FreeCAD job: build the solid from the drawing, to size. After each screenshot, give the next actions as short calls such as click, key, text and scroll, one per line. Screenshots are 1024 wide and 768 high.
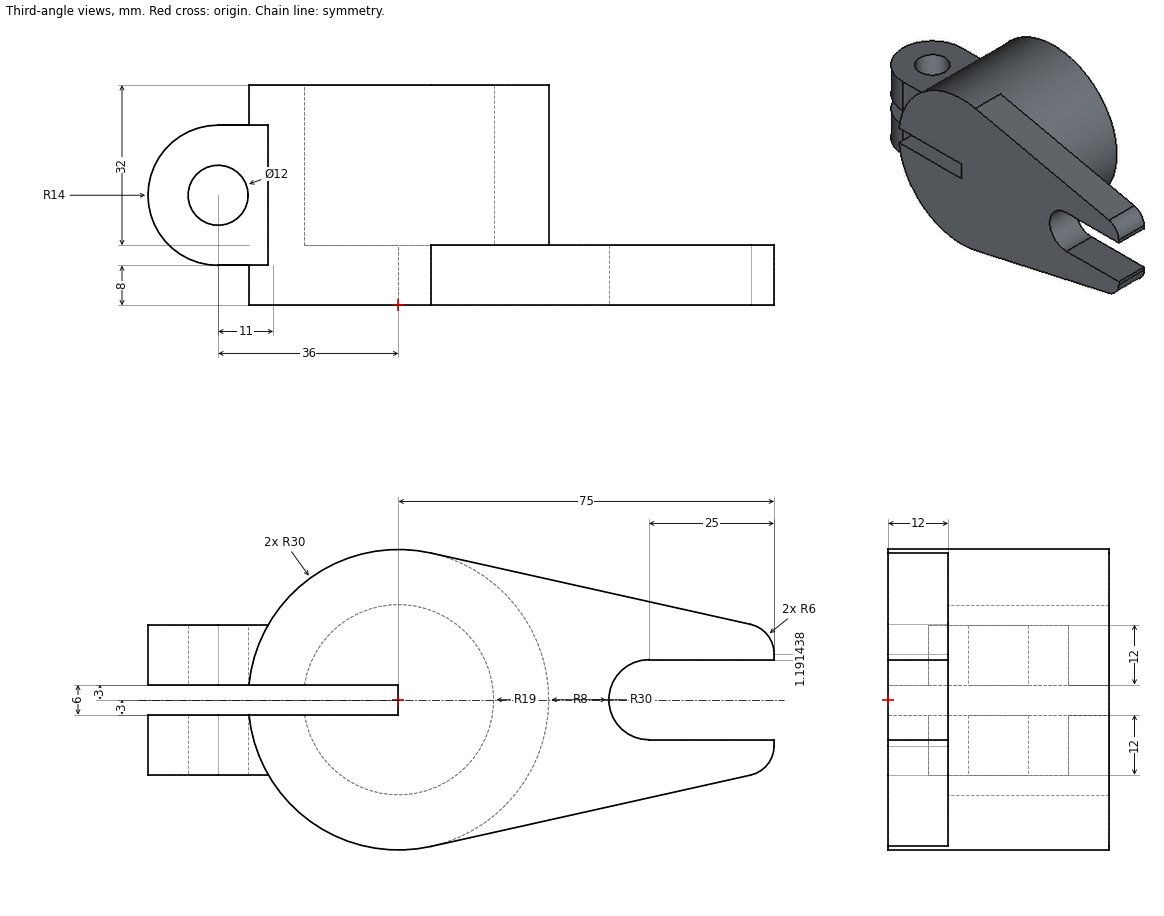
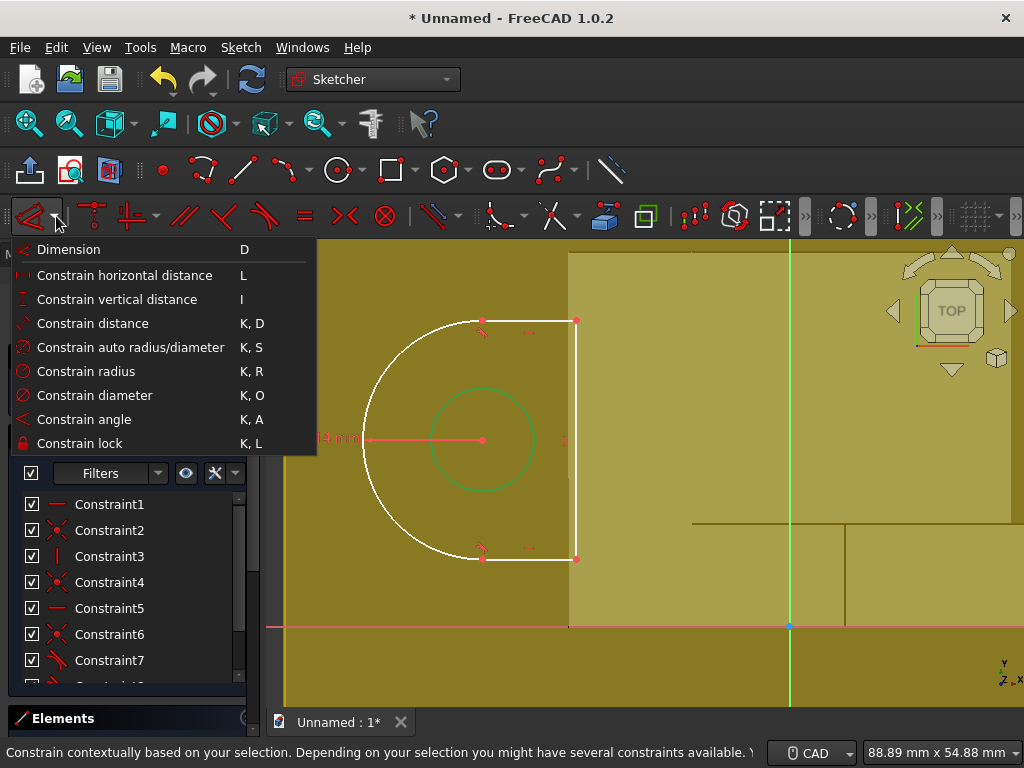
click(164, 395)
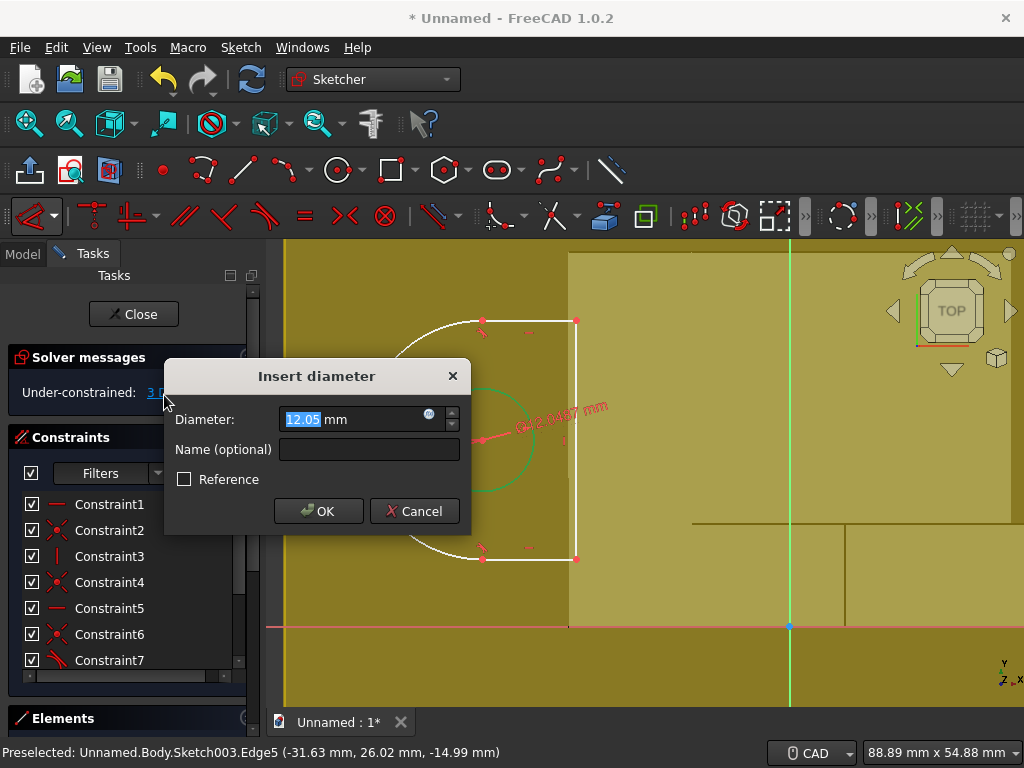
text(12)
key(Return)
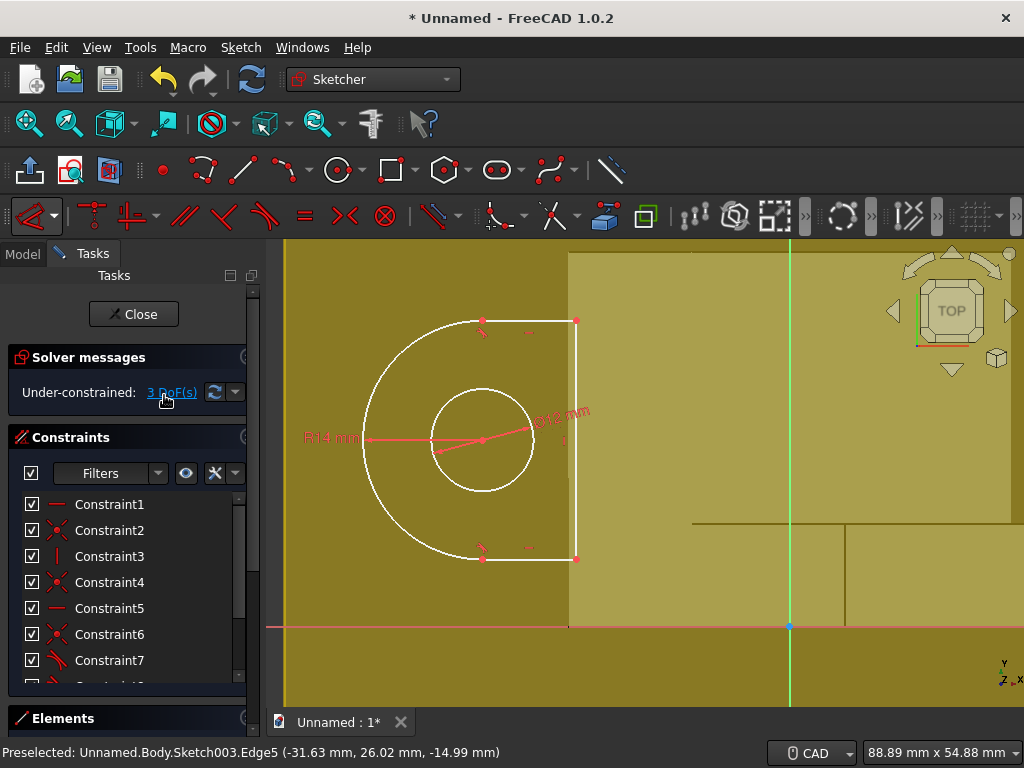
click(511, 560)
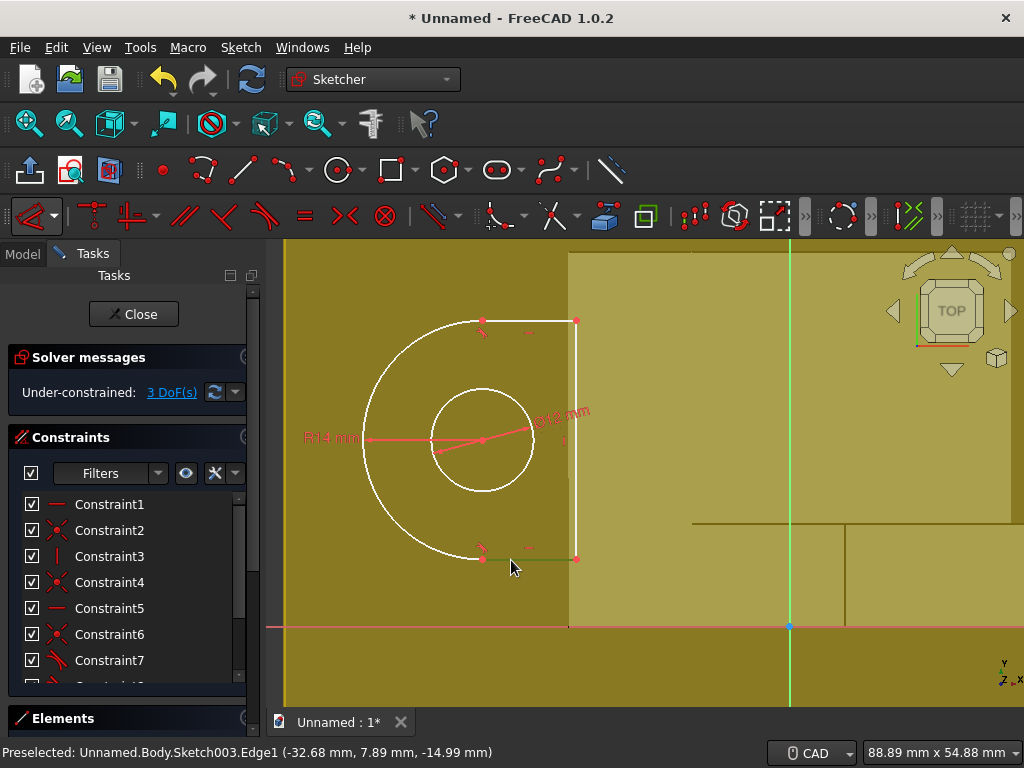
key(l)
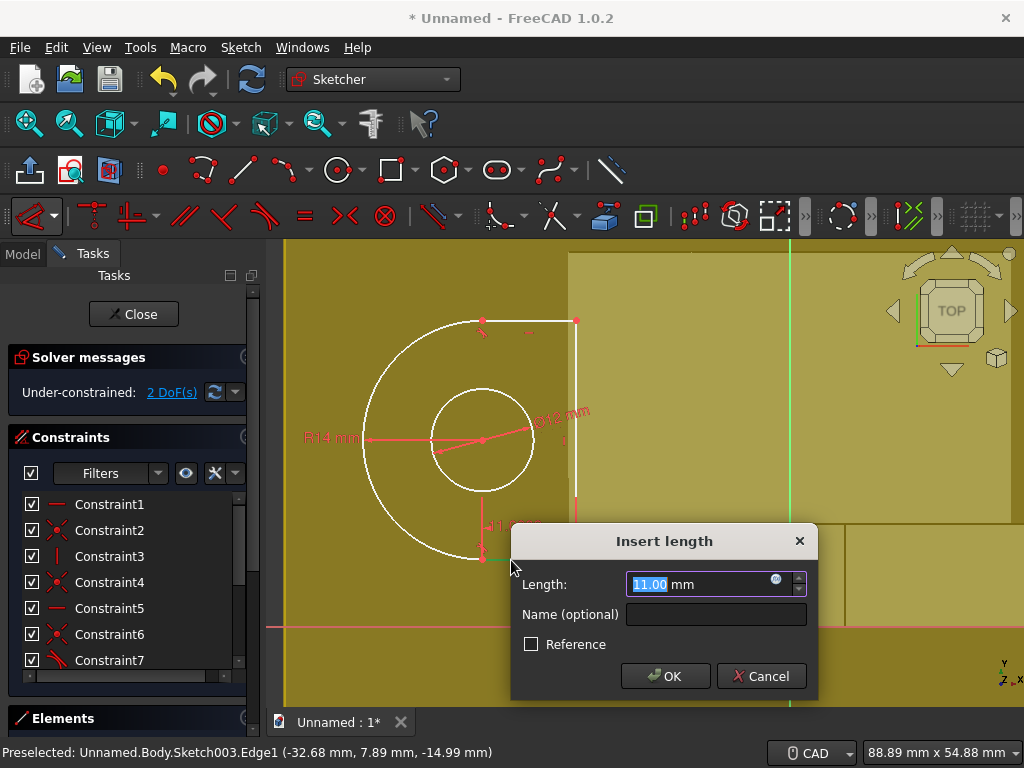
text(11)
key(Return)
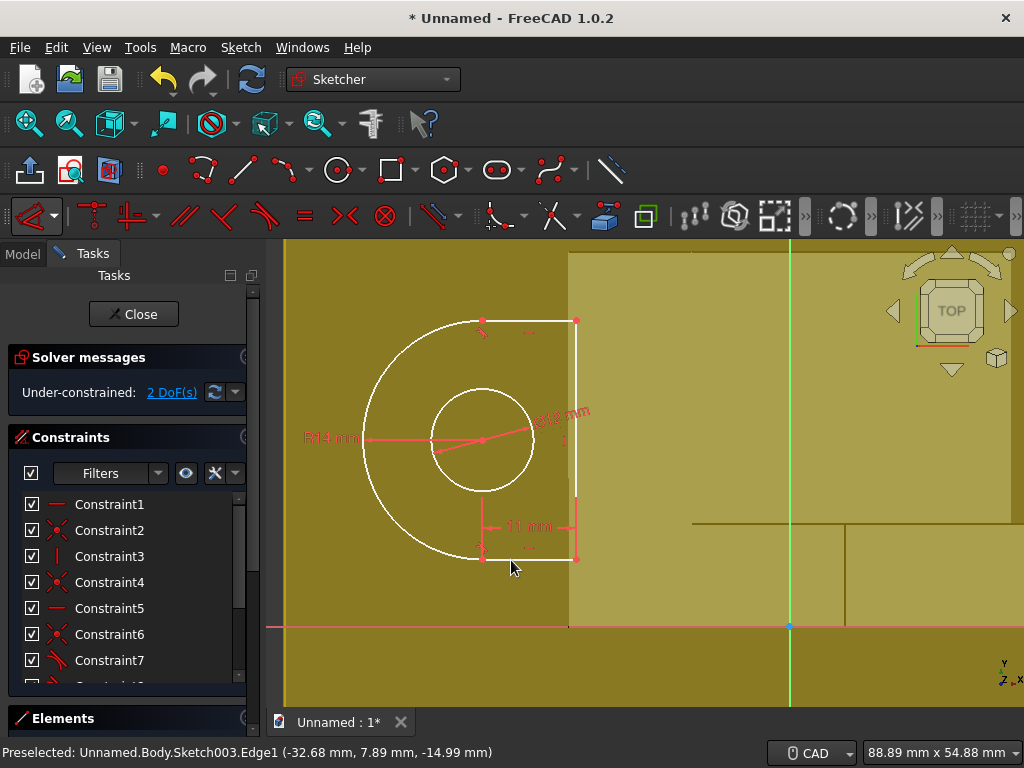
click(482, 560)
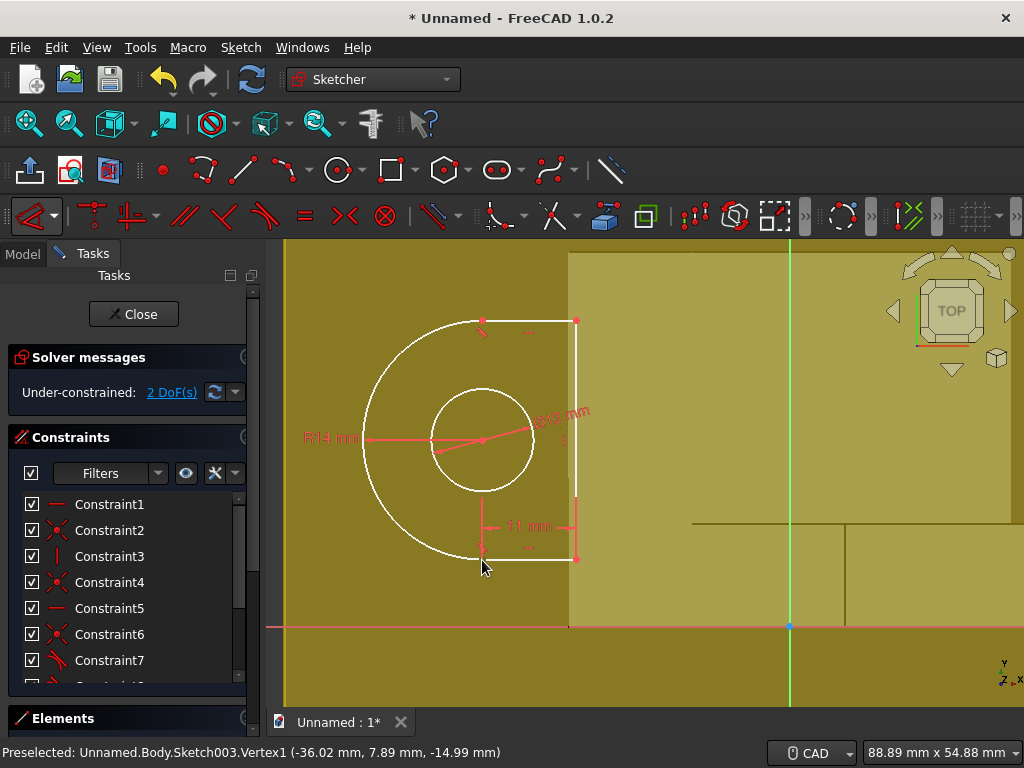
key(i)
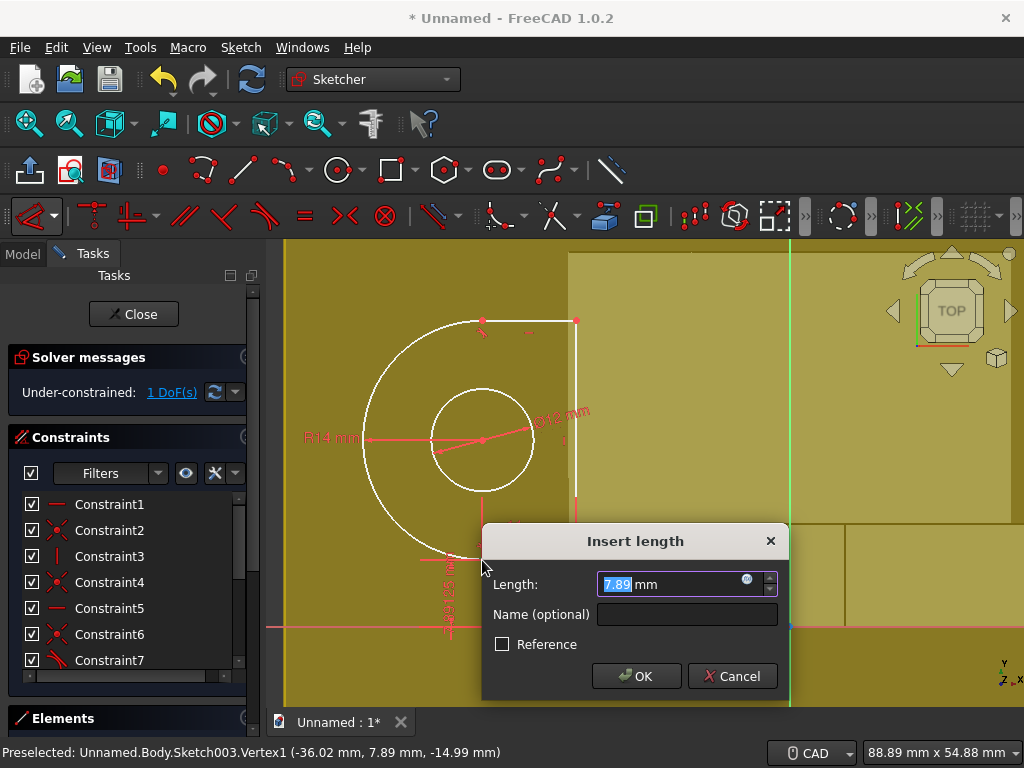
text(8)
key(Return)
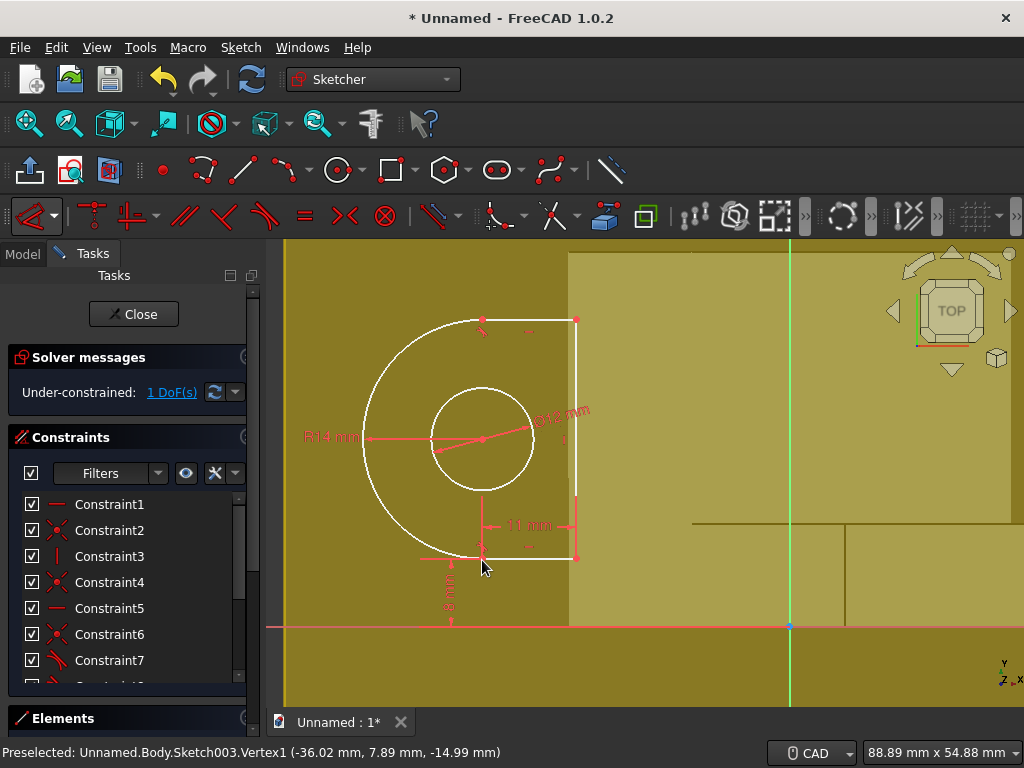
click(482, 439)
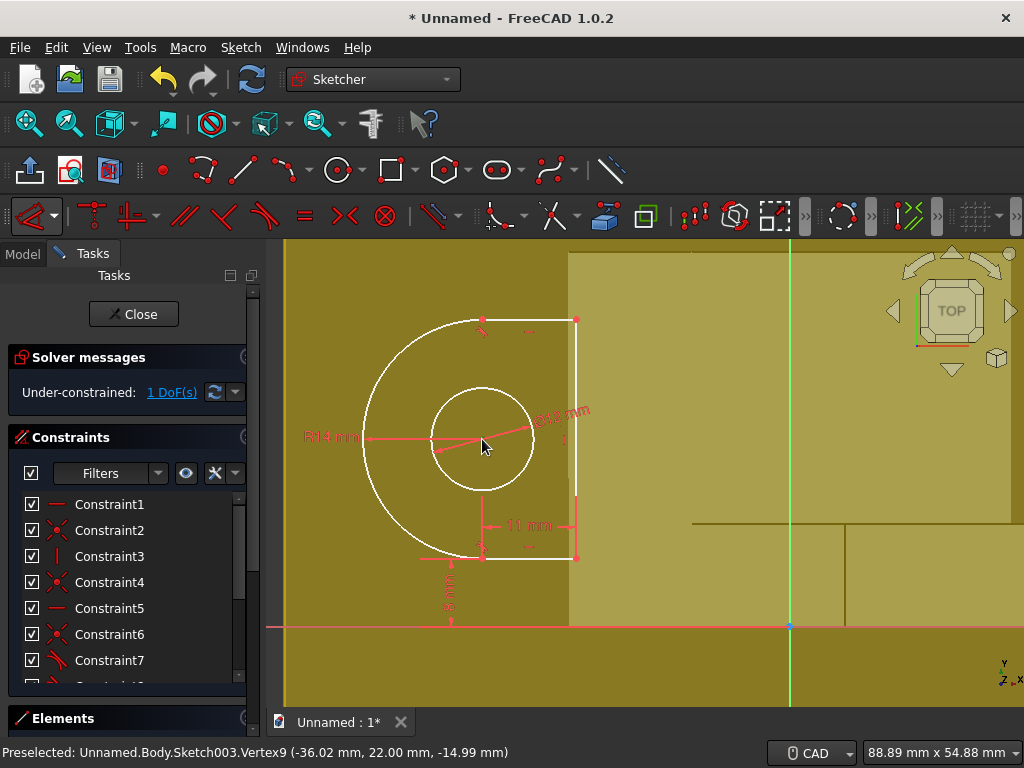
key(l)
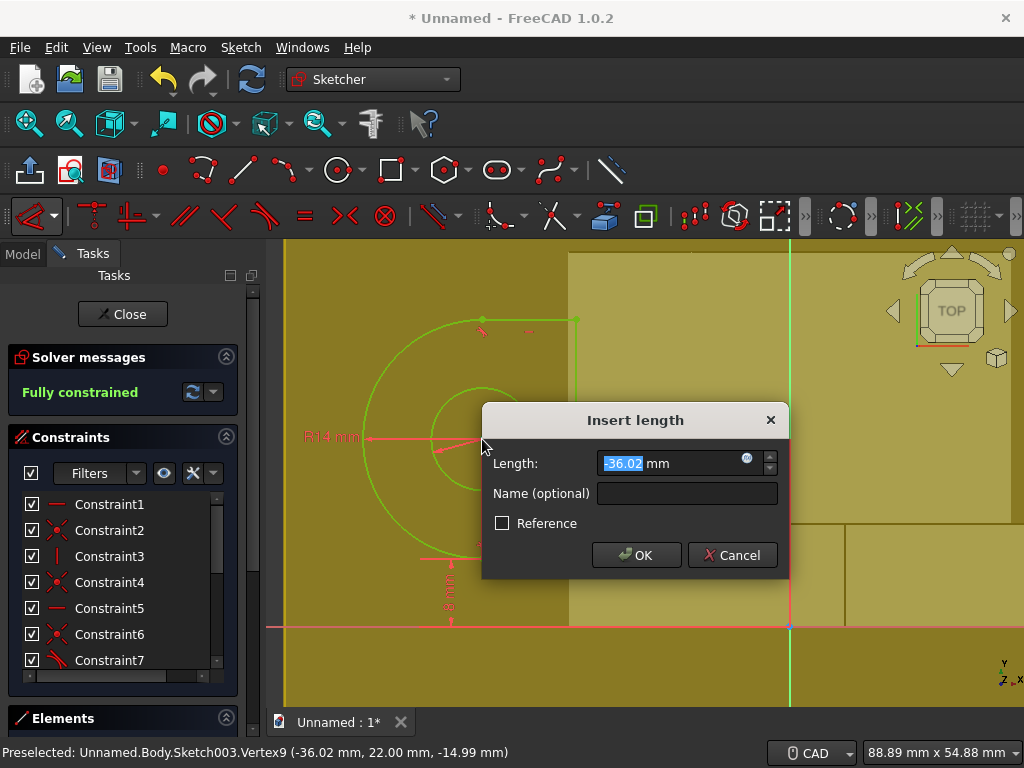
text(-36)
key(Return)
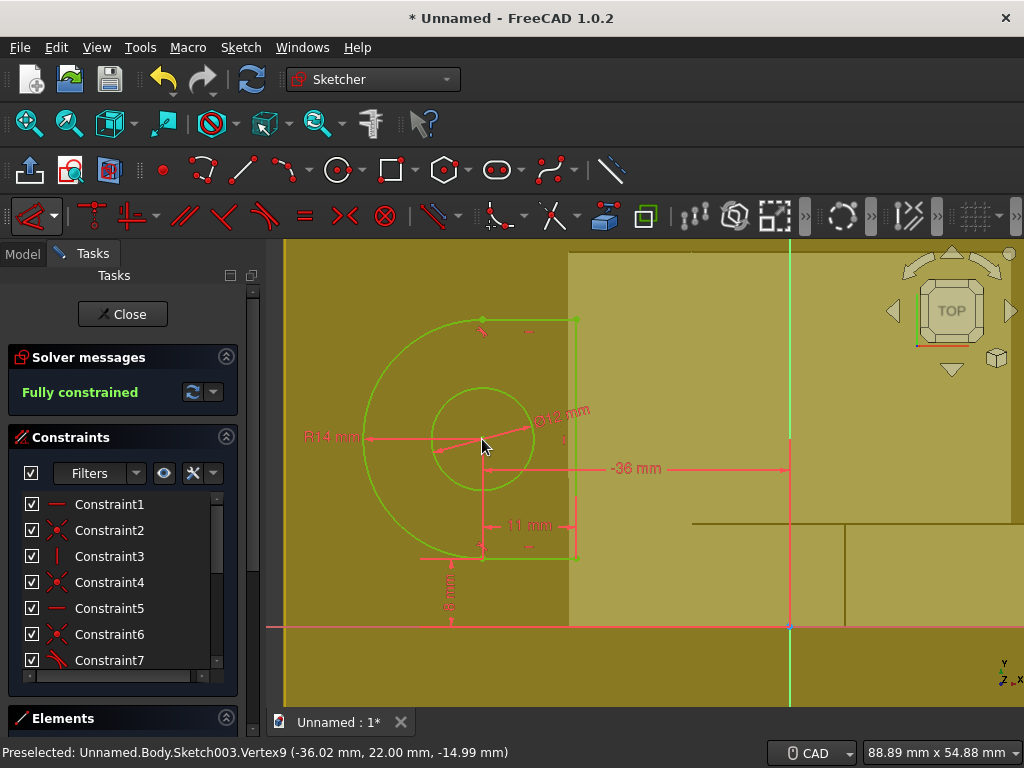
click(123, 314)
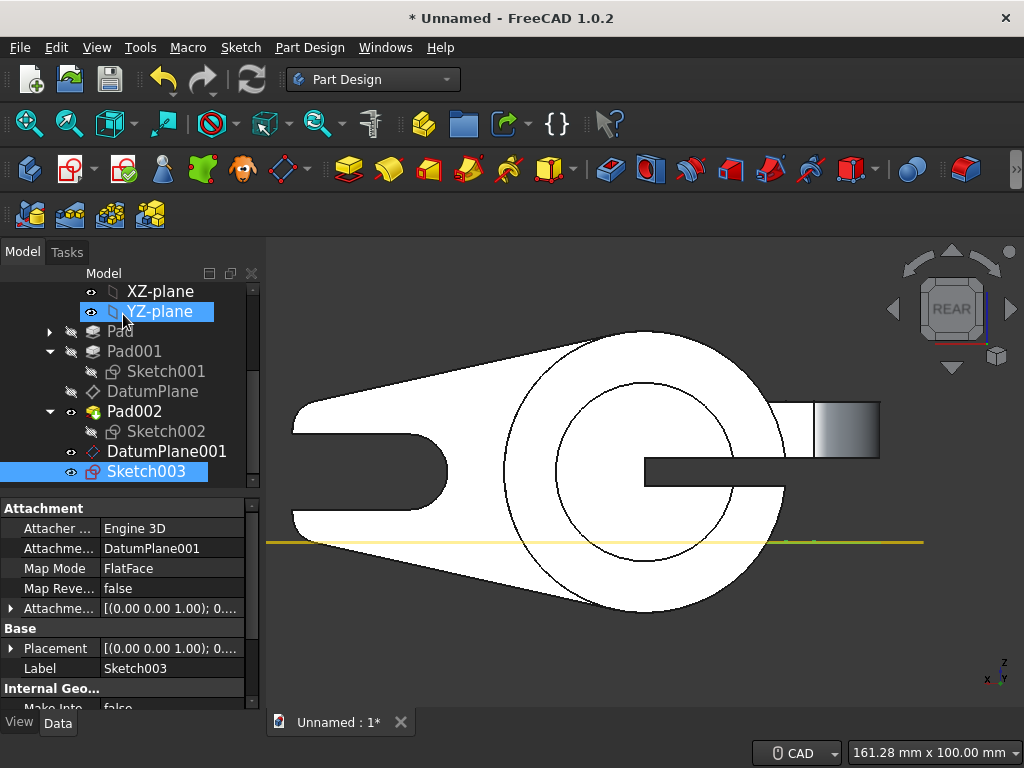
click(350, 170)